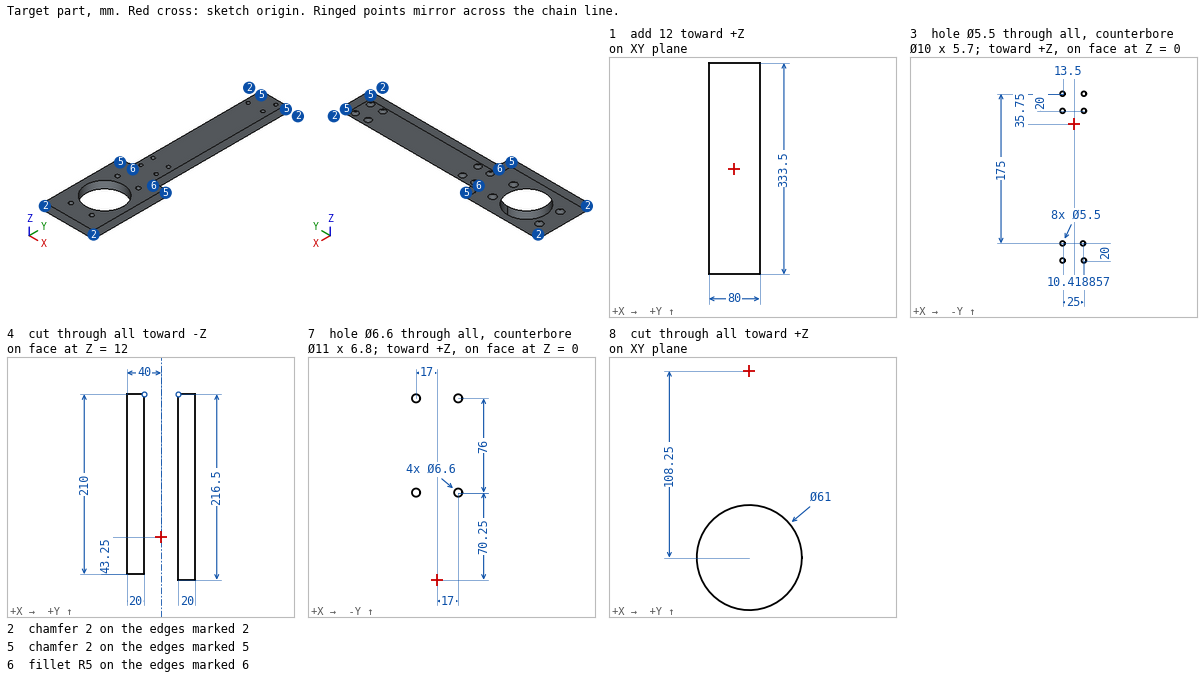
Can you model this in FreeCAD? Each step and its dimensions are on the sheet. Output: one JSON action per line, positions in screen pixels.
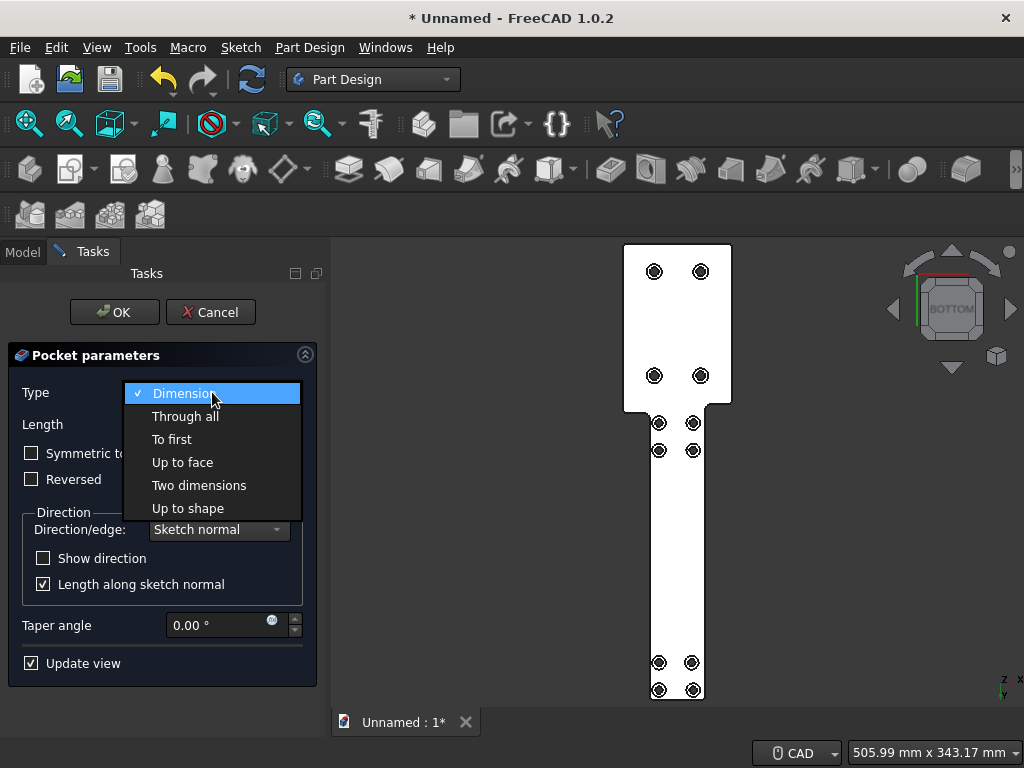
{"action": "left_click", "coordinate": [212, 416]}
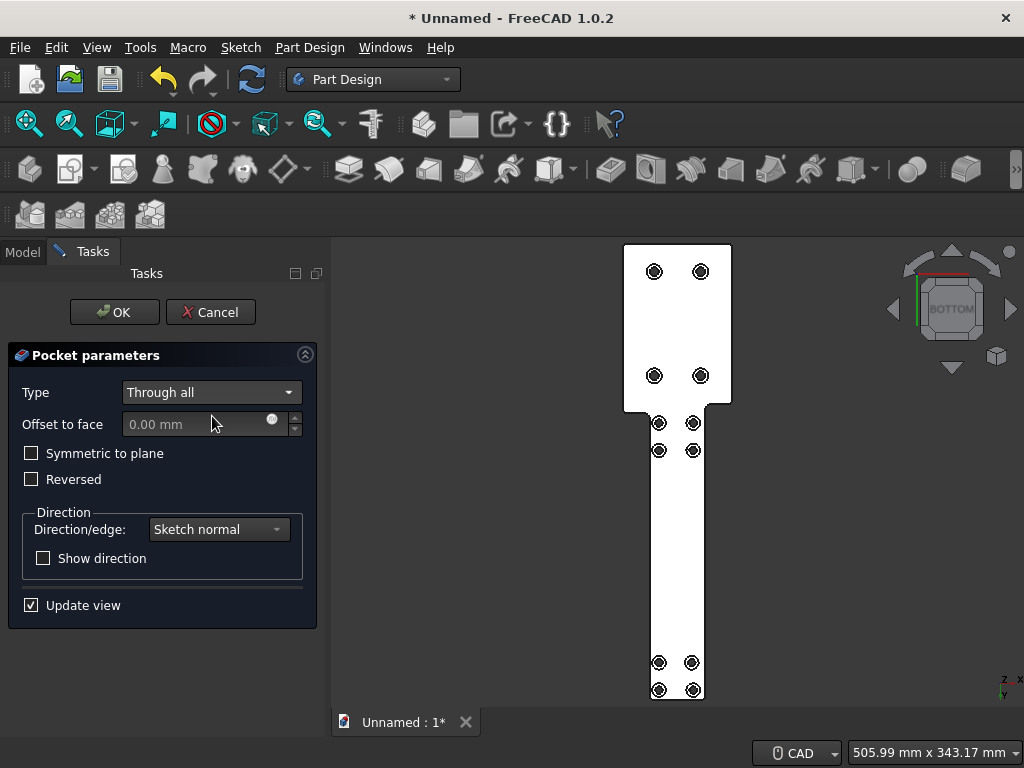
{"action": "left_click", "coordinate": [30, 479]}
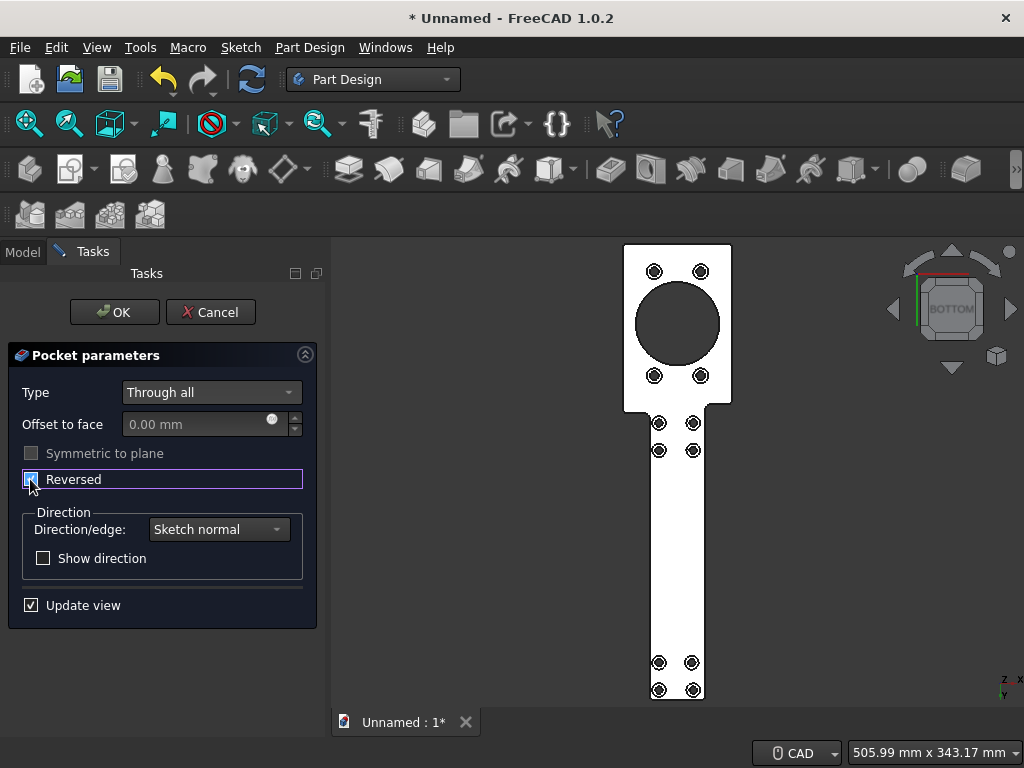
{"action": "left_click", "coordinate": [115, 312]}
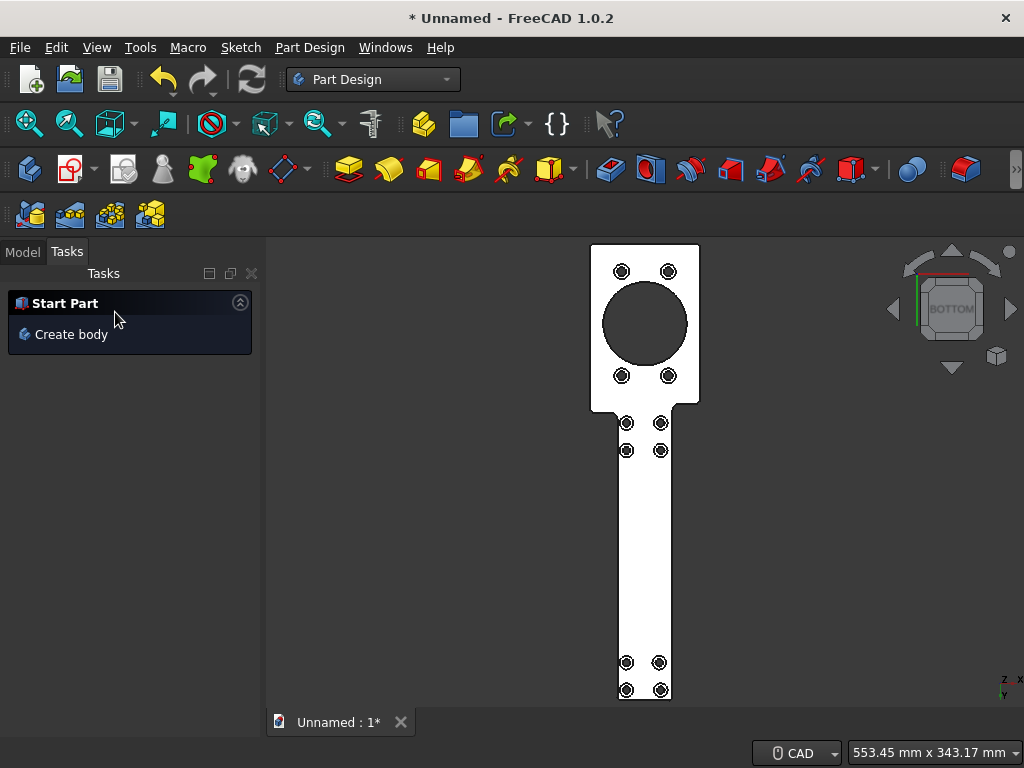
{"action": "key", "text": "0"}